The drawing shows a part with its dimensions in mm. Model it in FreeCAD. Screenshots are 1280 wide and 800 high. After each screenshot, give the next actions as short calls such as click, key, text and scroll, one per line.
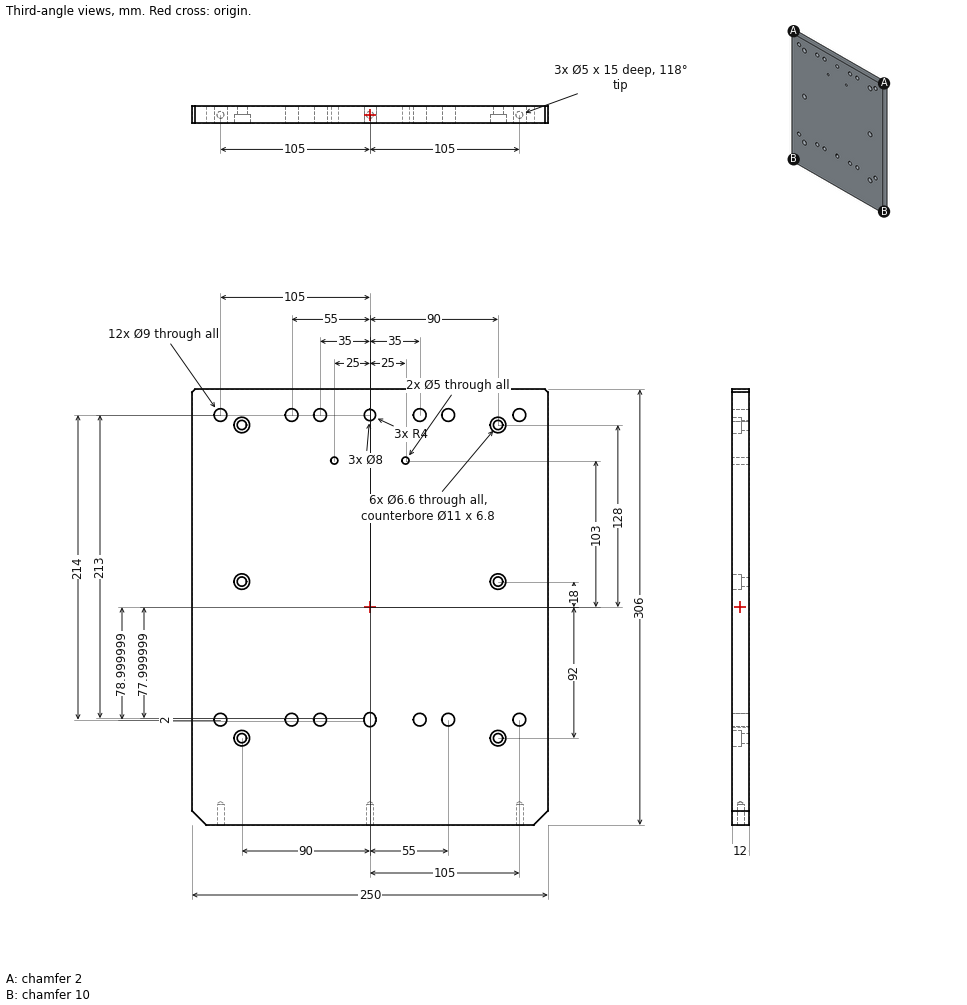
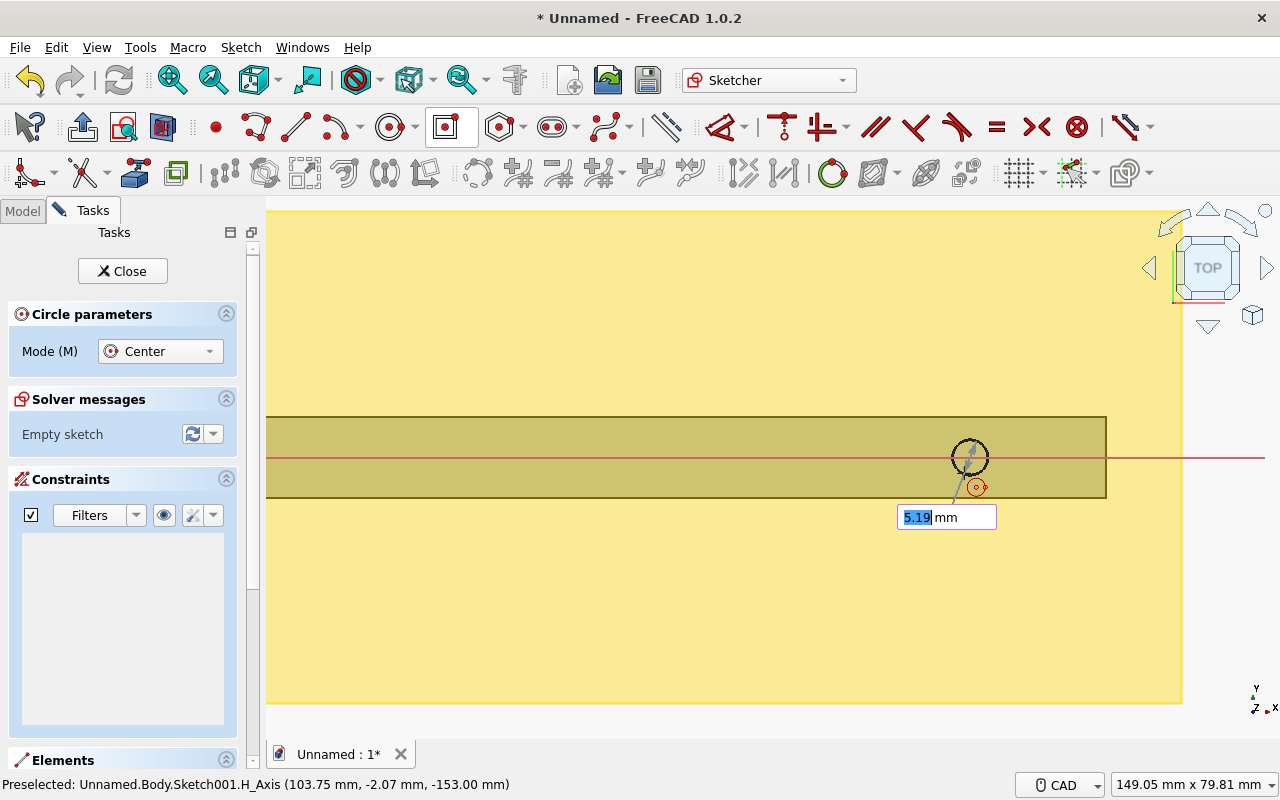
text(5)
key(Return)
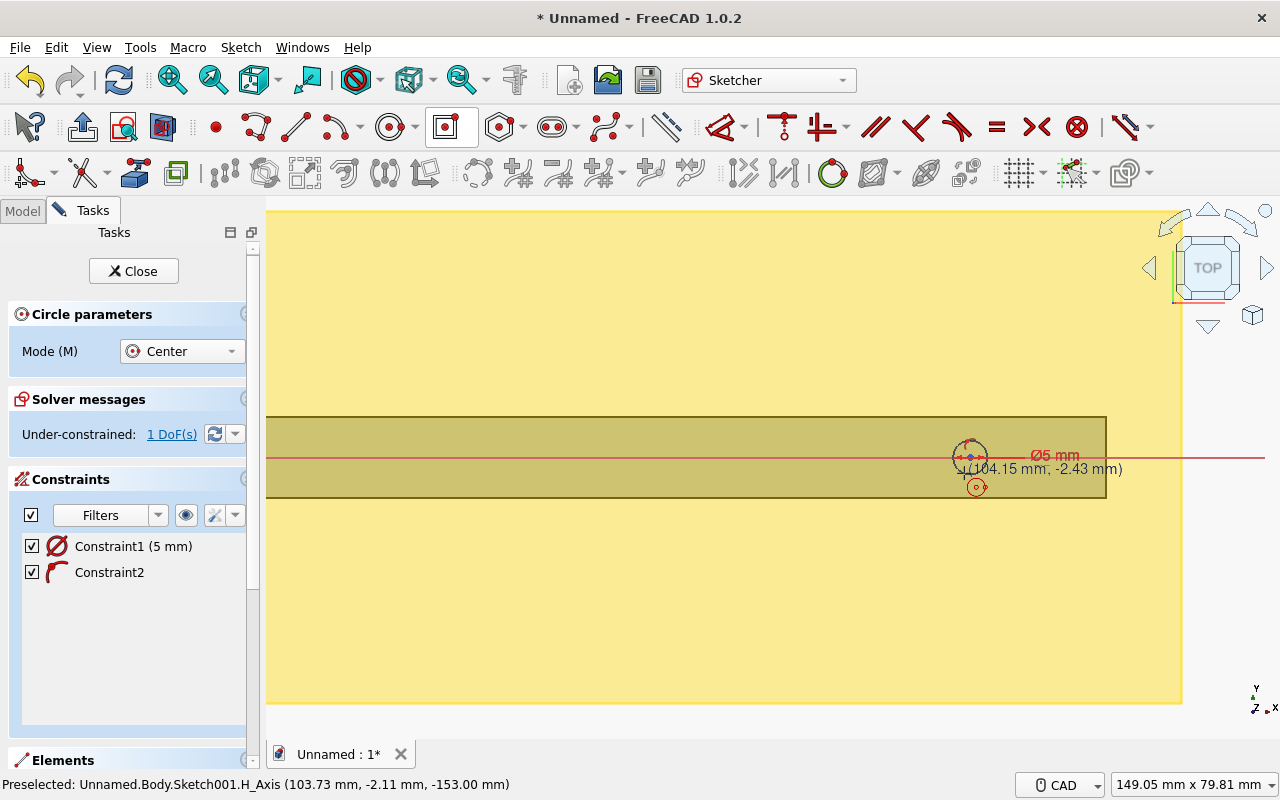
scroll(966, 473, down, 5)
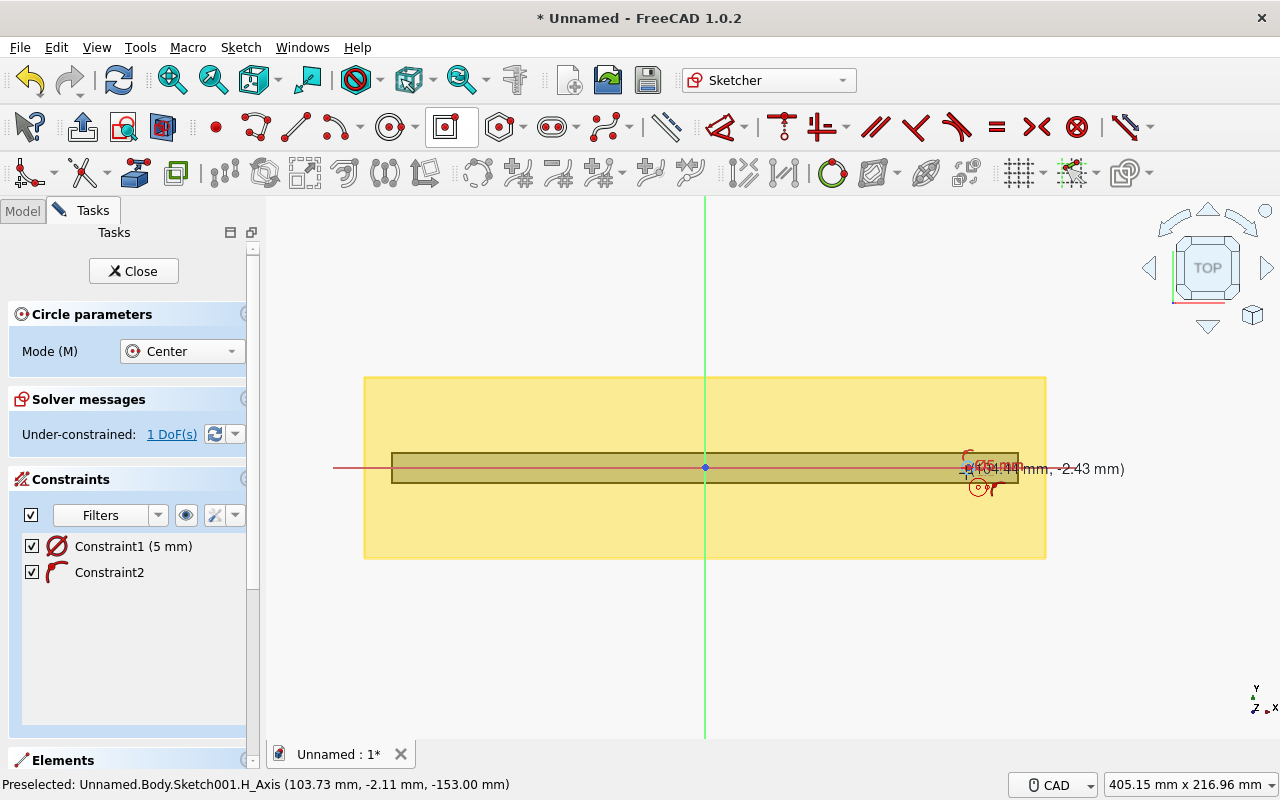
scroll(705, 468, up, 7)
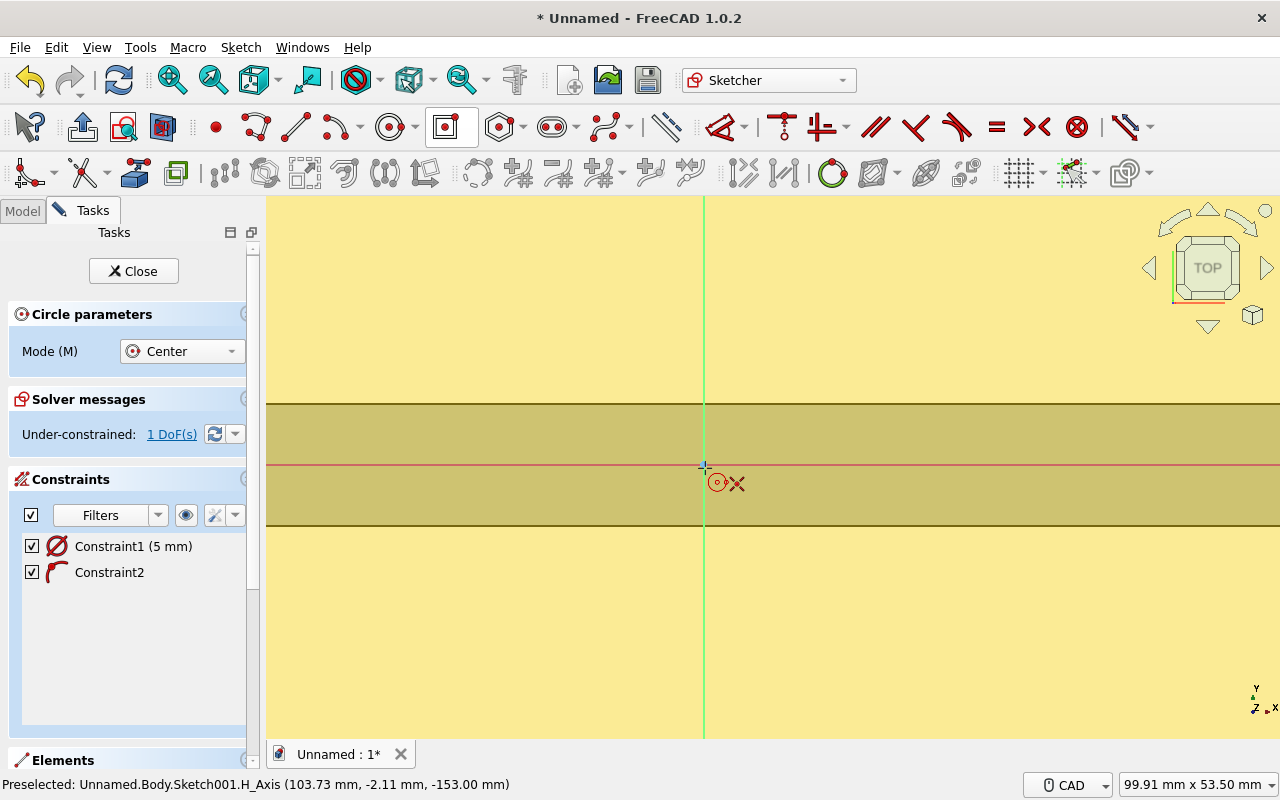
scroll(705, 468, down, 7)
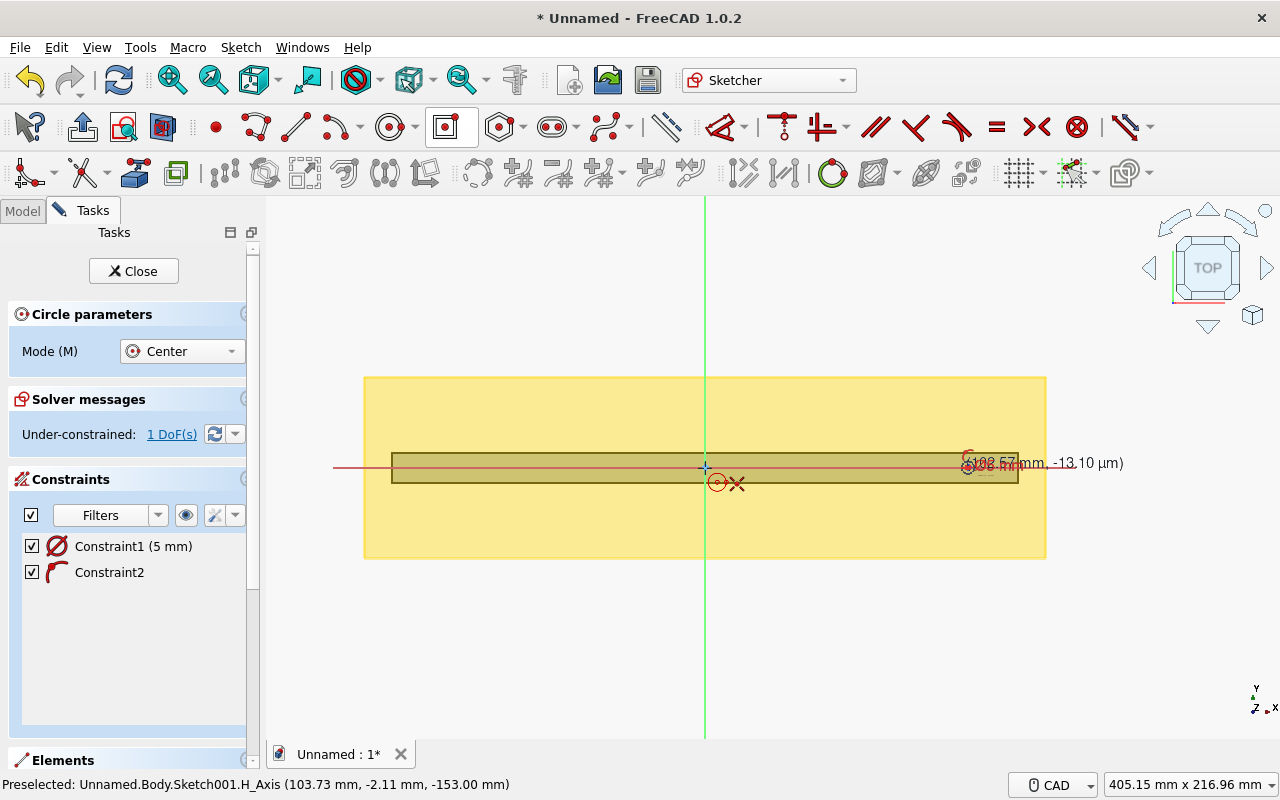
click(705, 468)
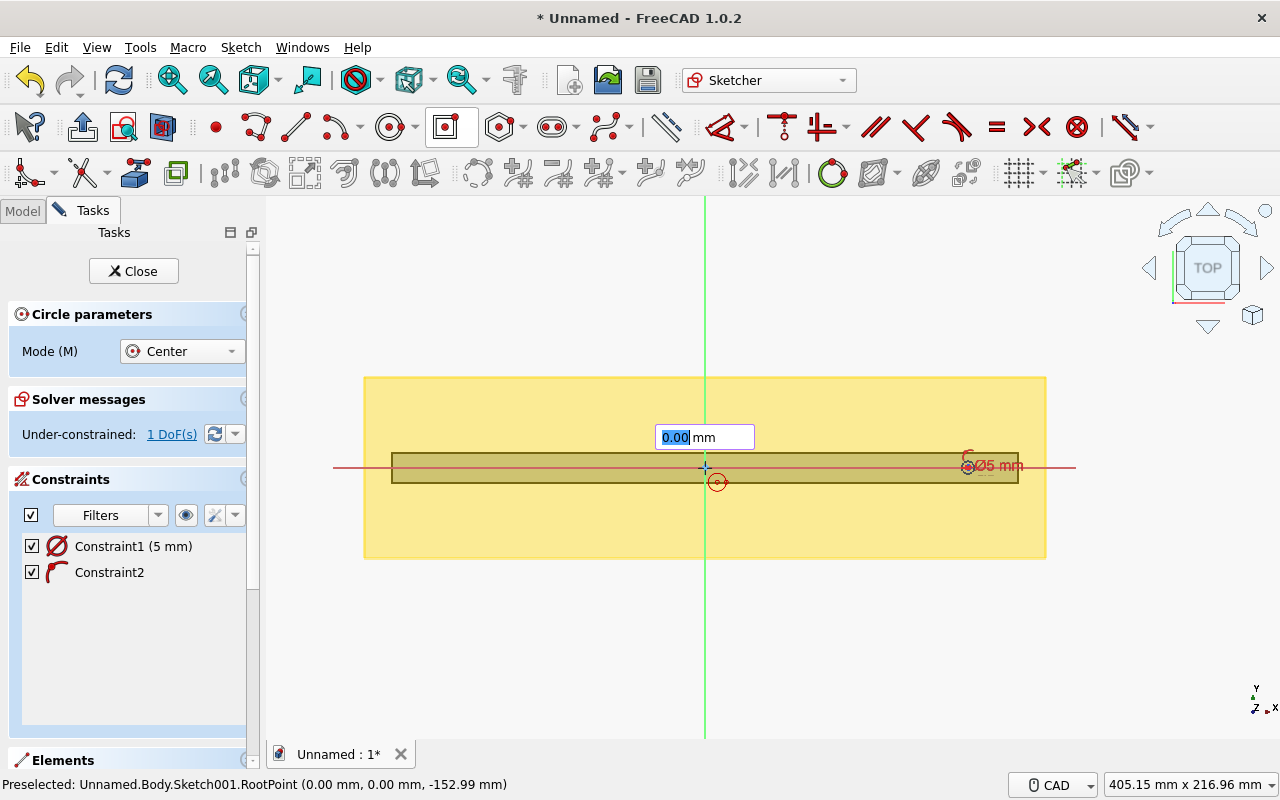
scroll(709, 463, up, 7)
move(710, 462)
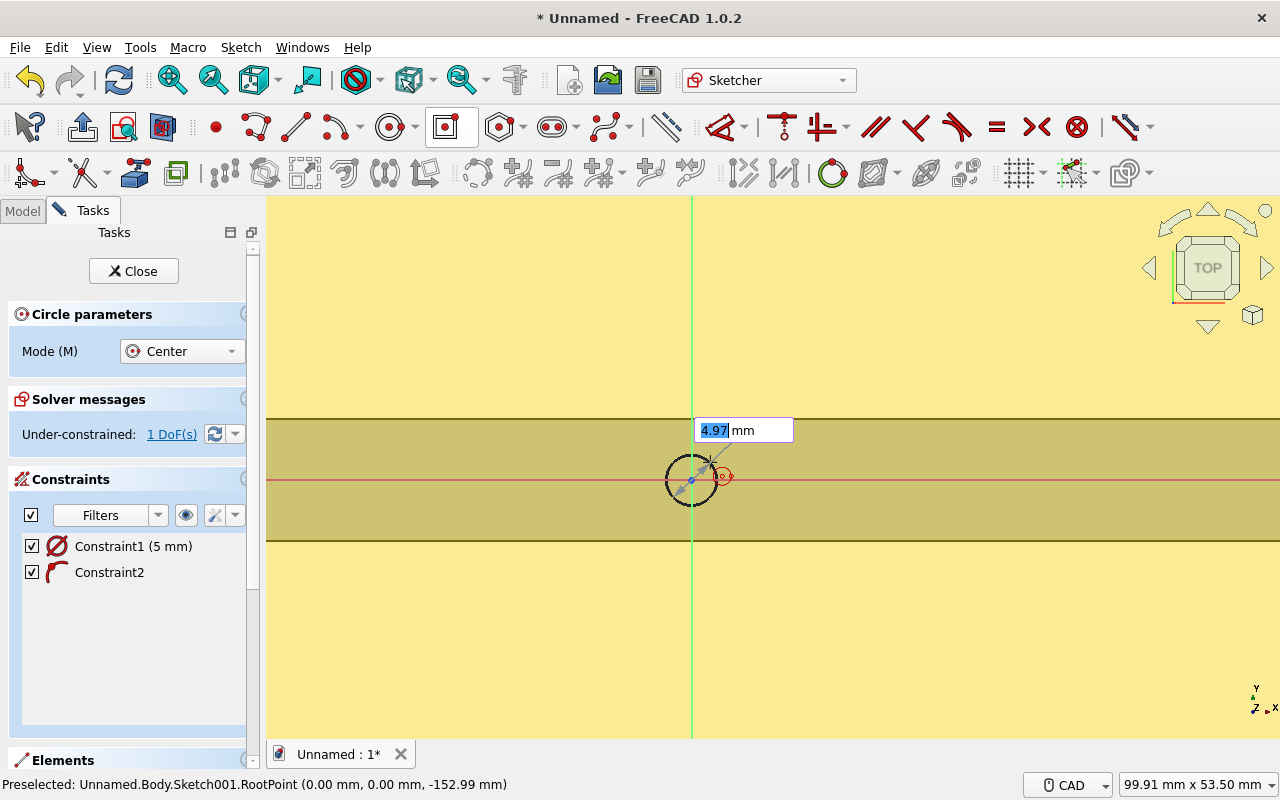
text(5)
key(Return)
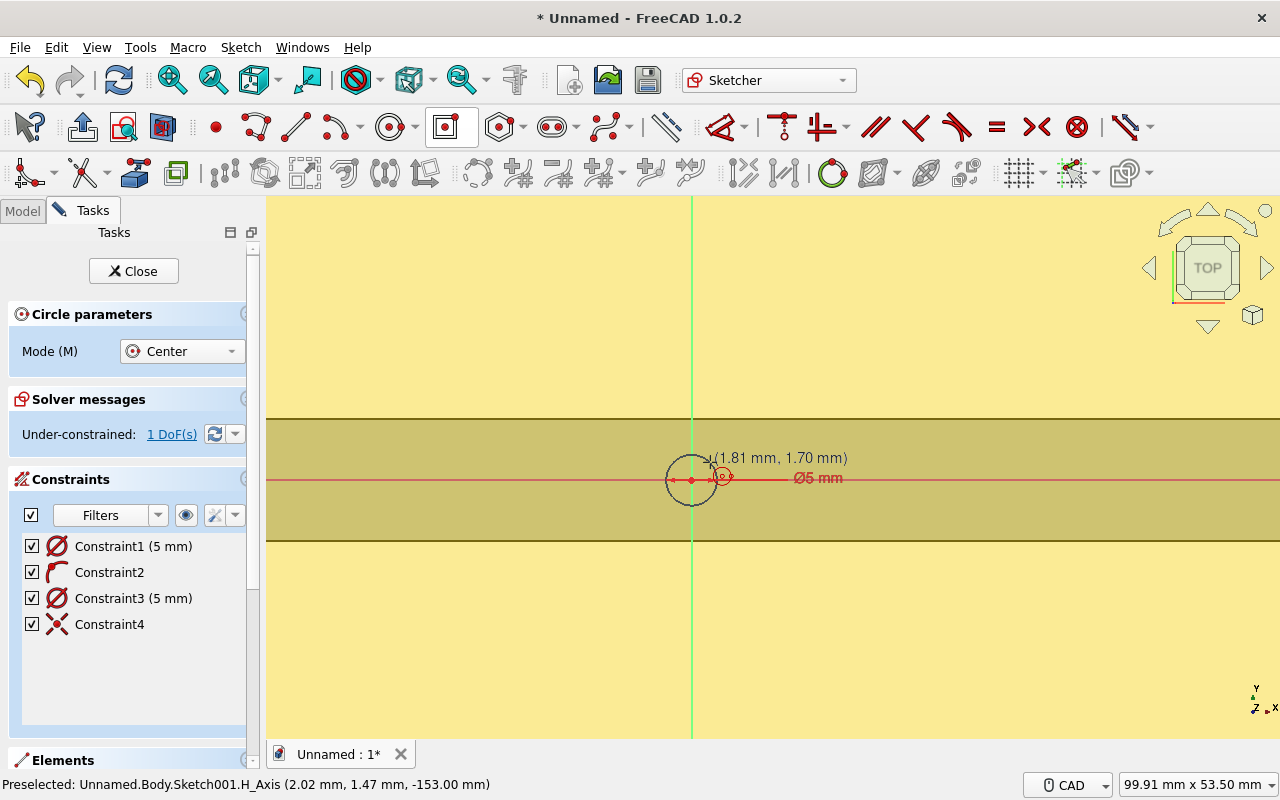
scroll(709, 463, down, 7)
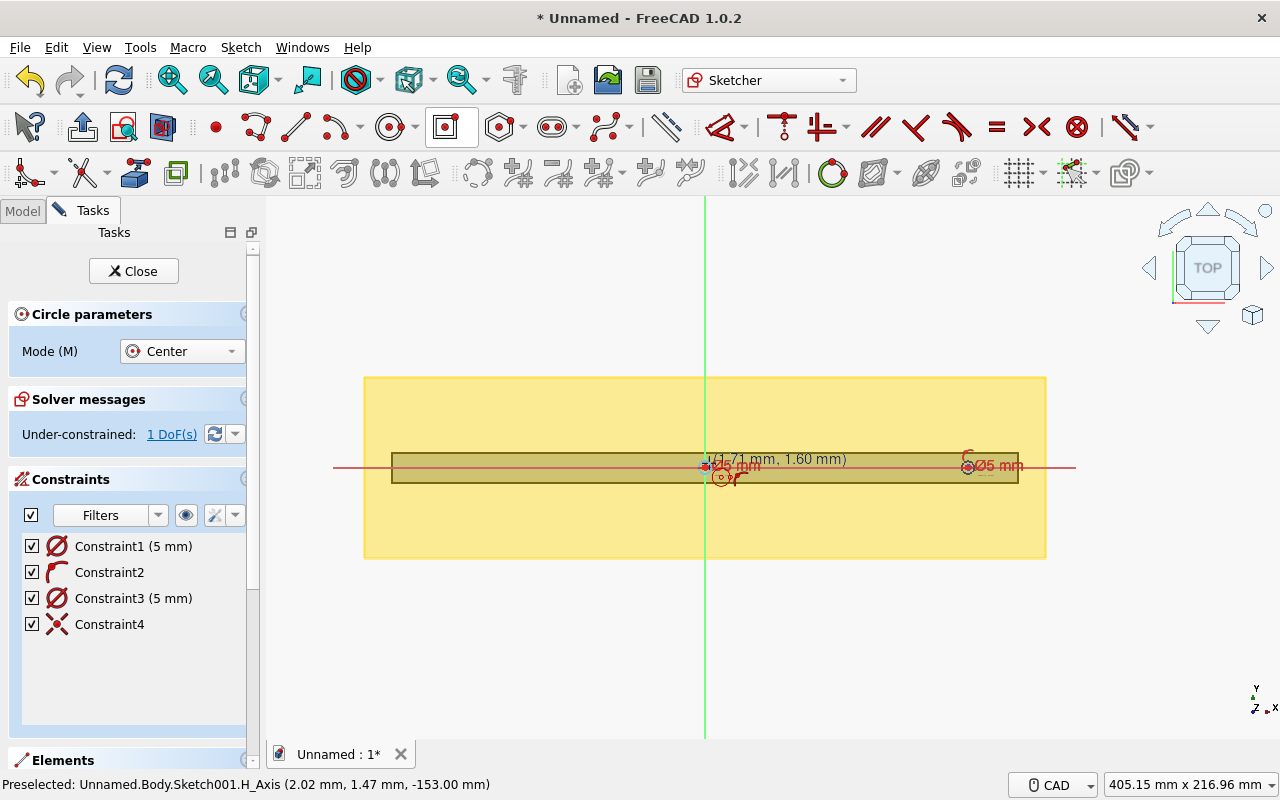
scroll(442, 468, up, 7)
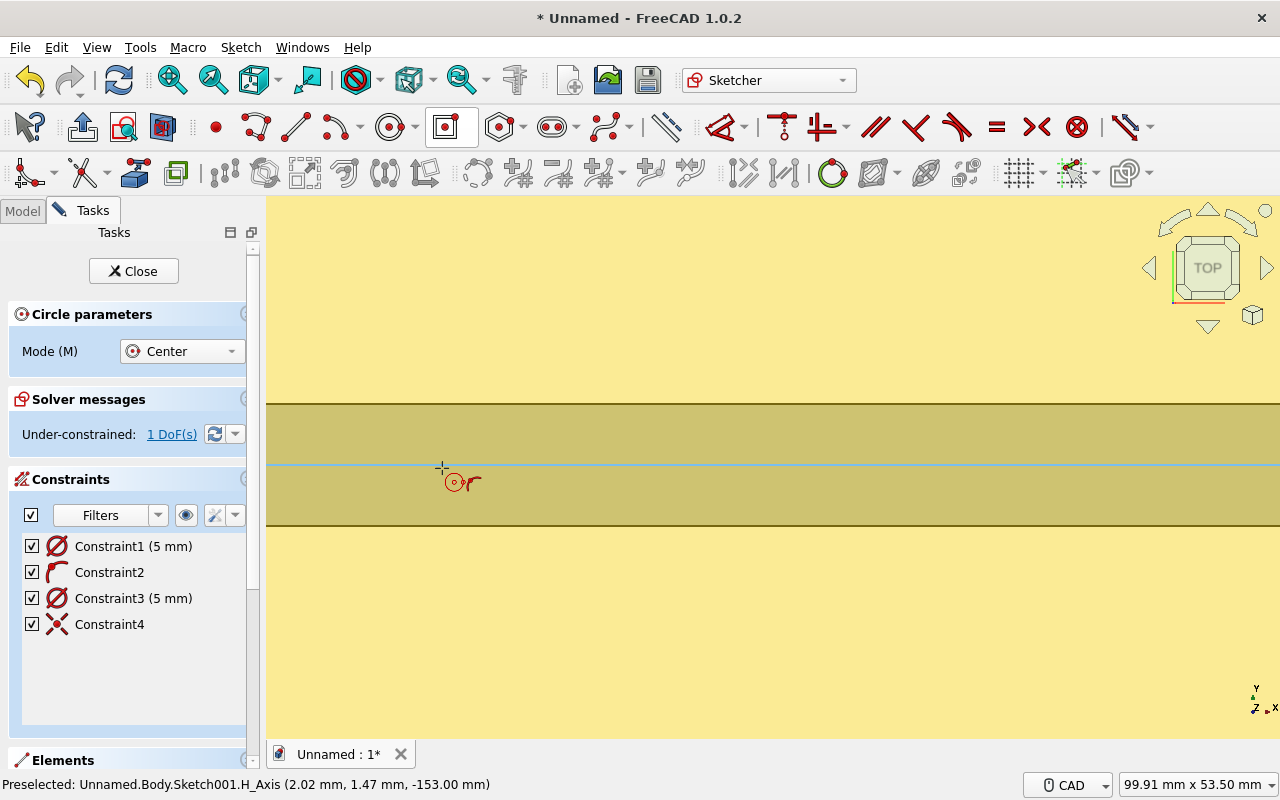
scroll(441, 468, down, 7)